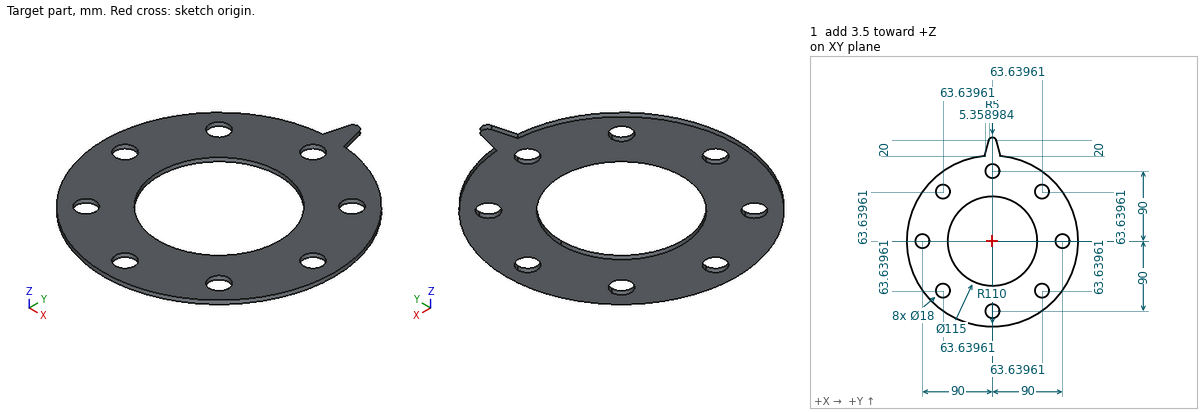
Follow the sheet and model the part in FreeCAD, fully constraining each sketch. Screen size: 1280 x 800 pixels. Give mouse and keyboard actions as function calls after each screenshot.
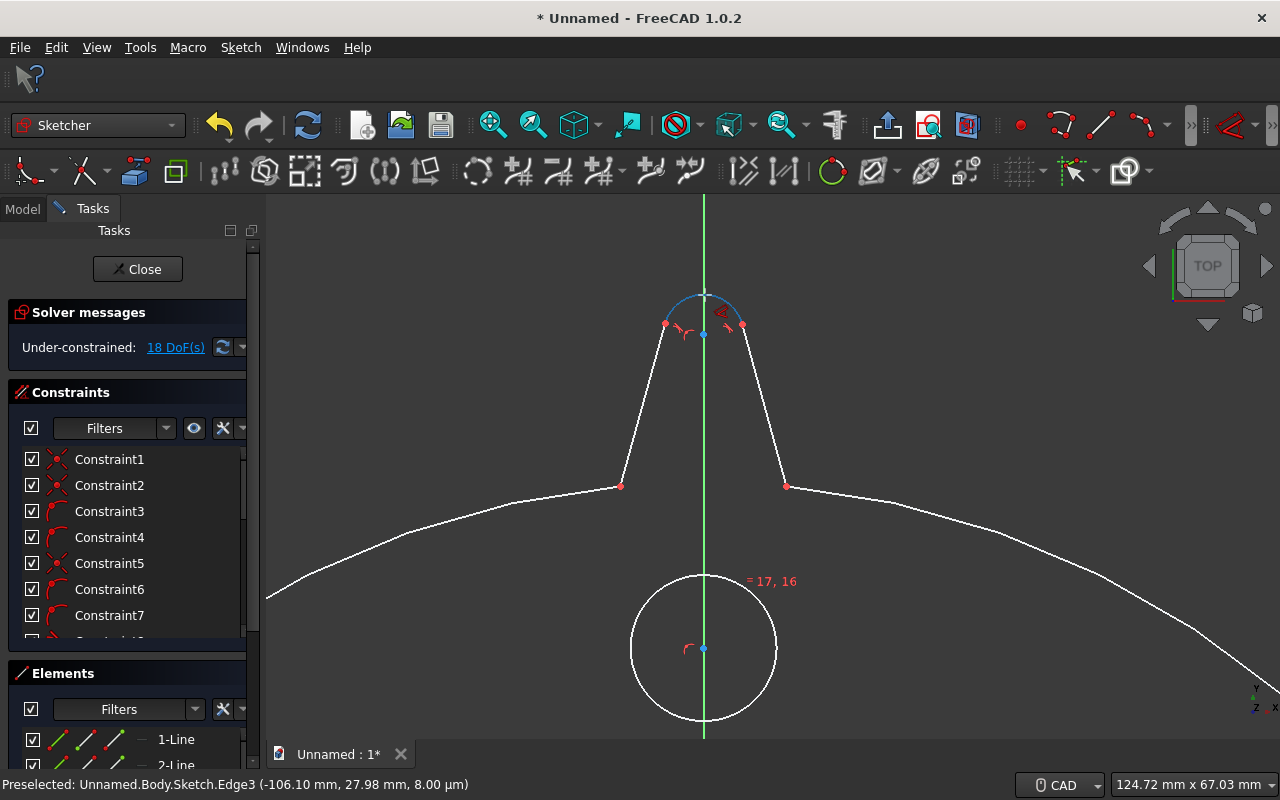
click(704, 295)
click(739, 272)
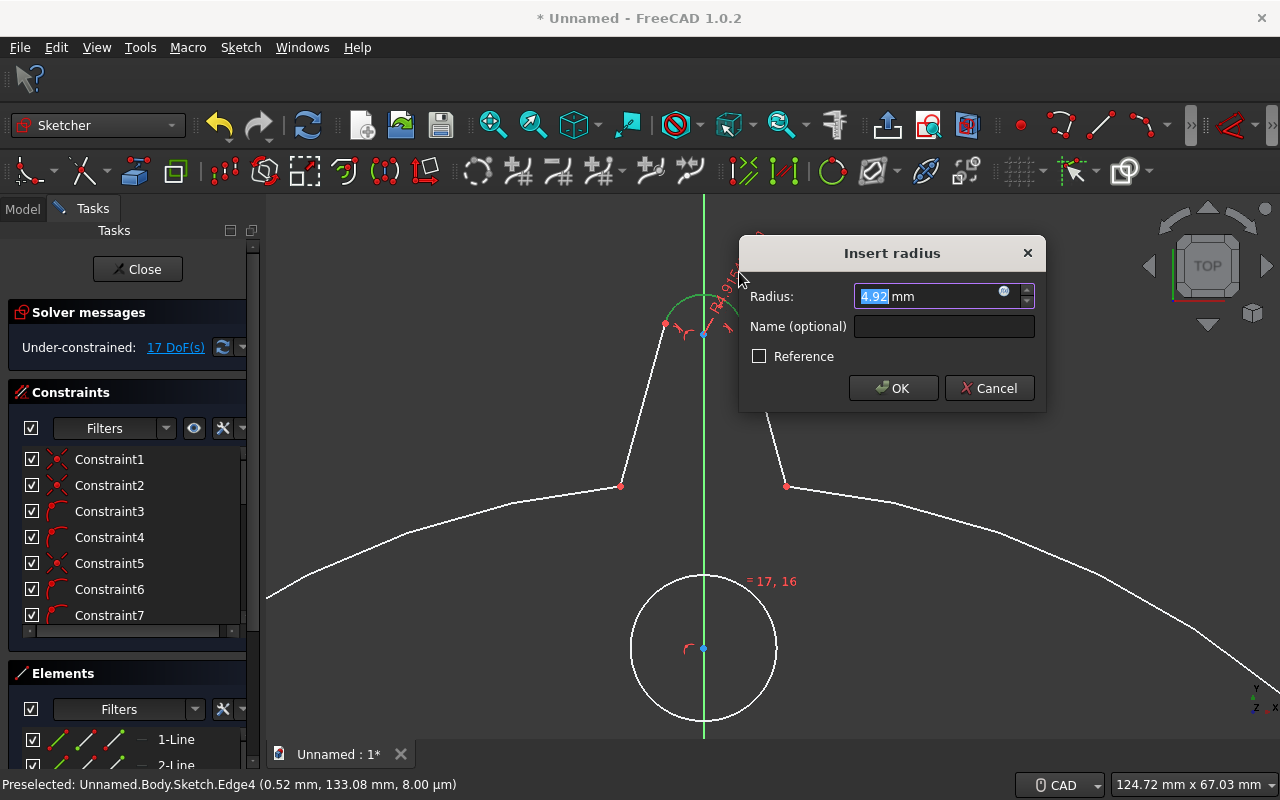
text(5)
key(Return)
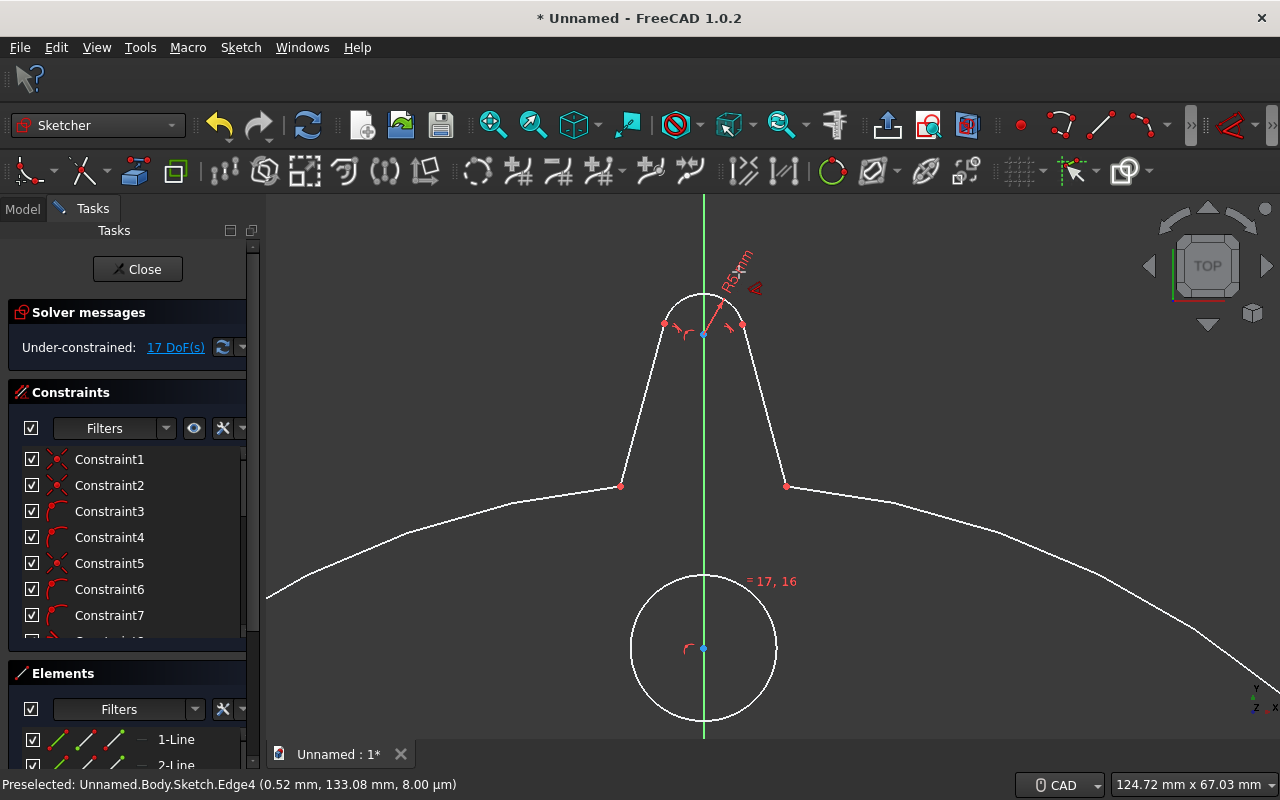
scroll(705, 305, down, 9)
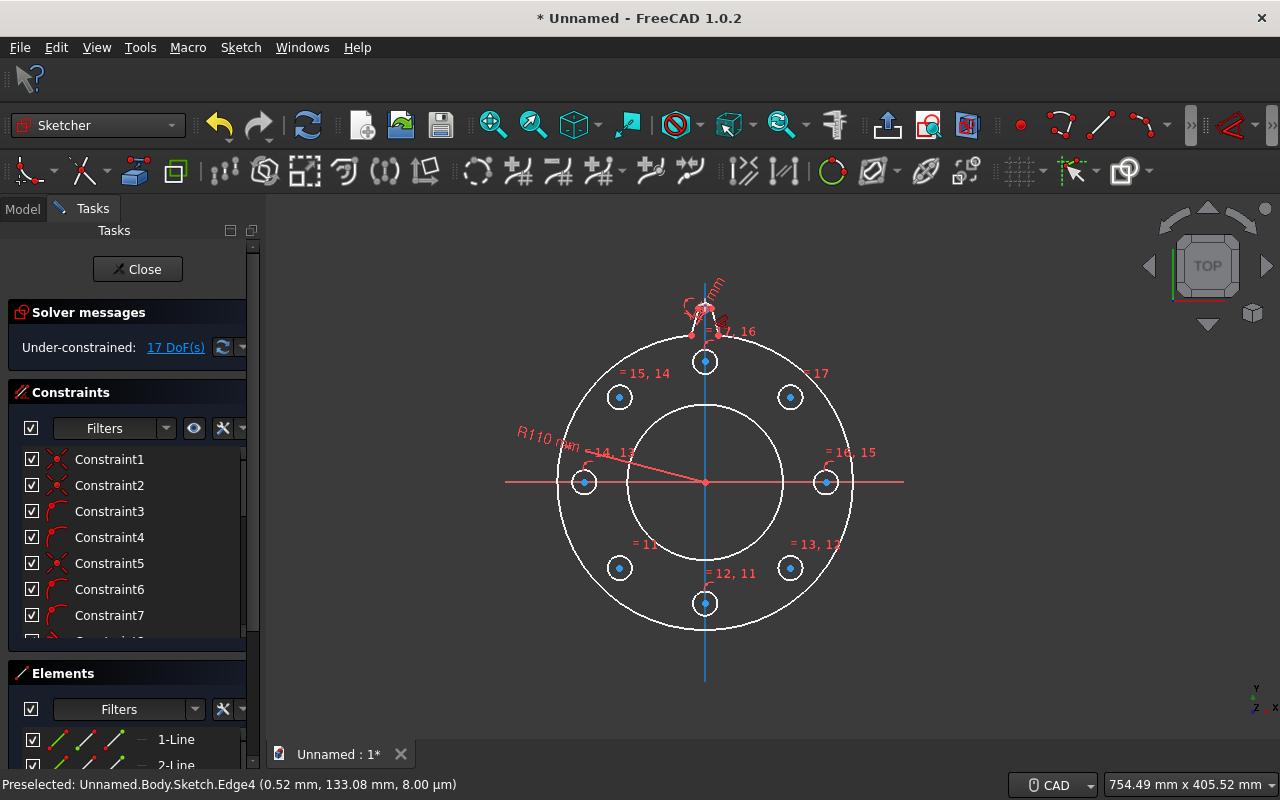
scroll(628, 560, up, 3)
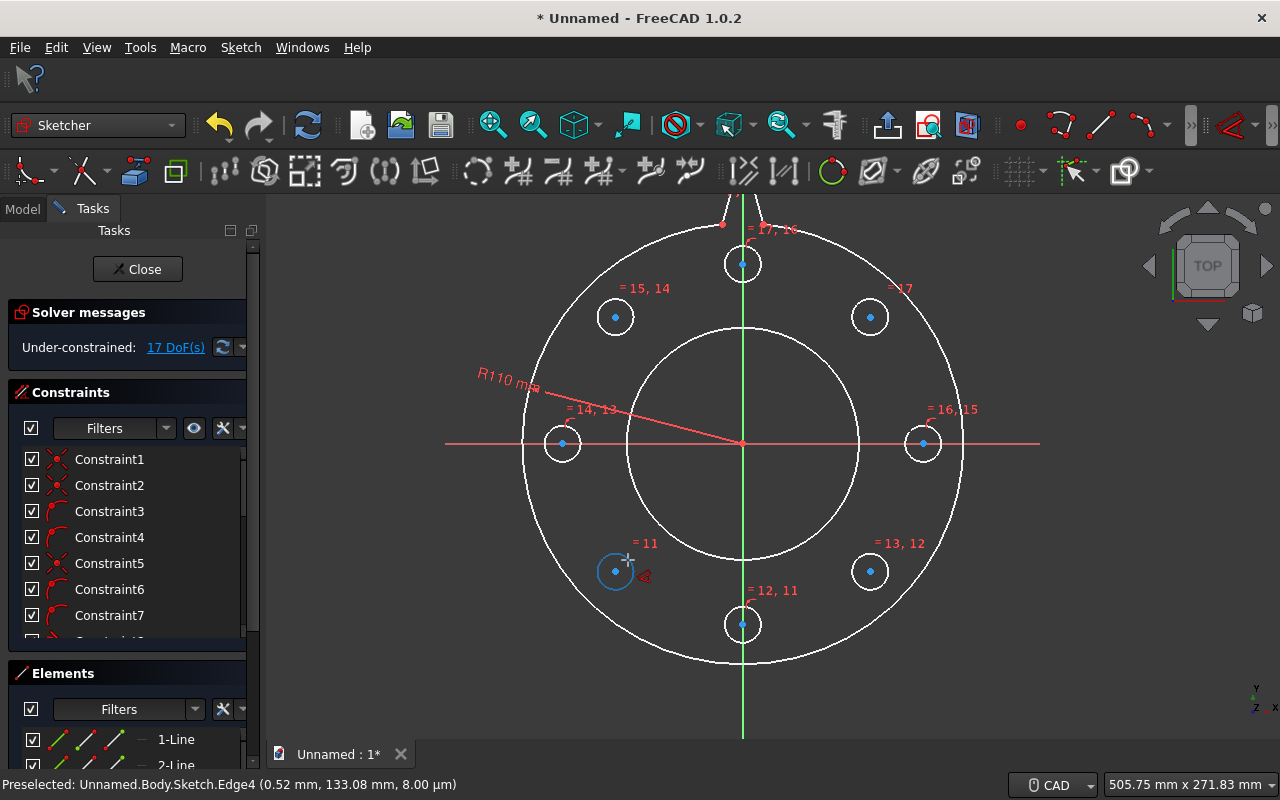
click(628, 559)
click(651, 536)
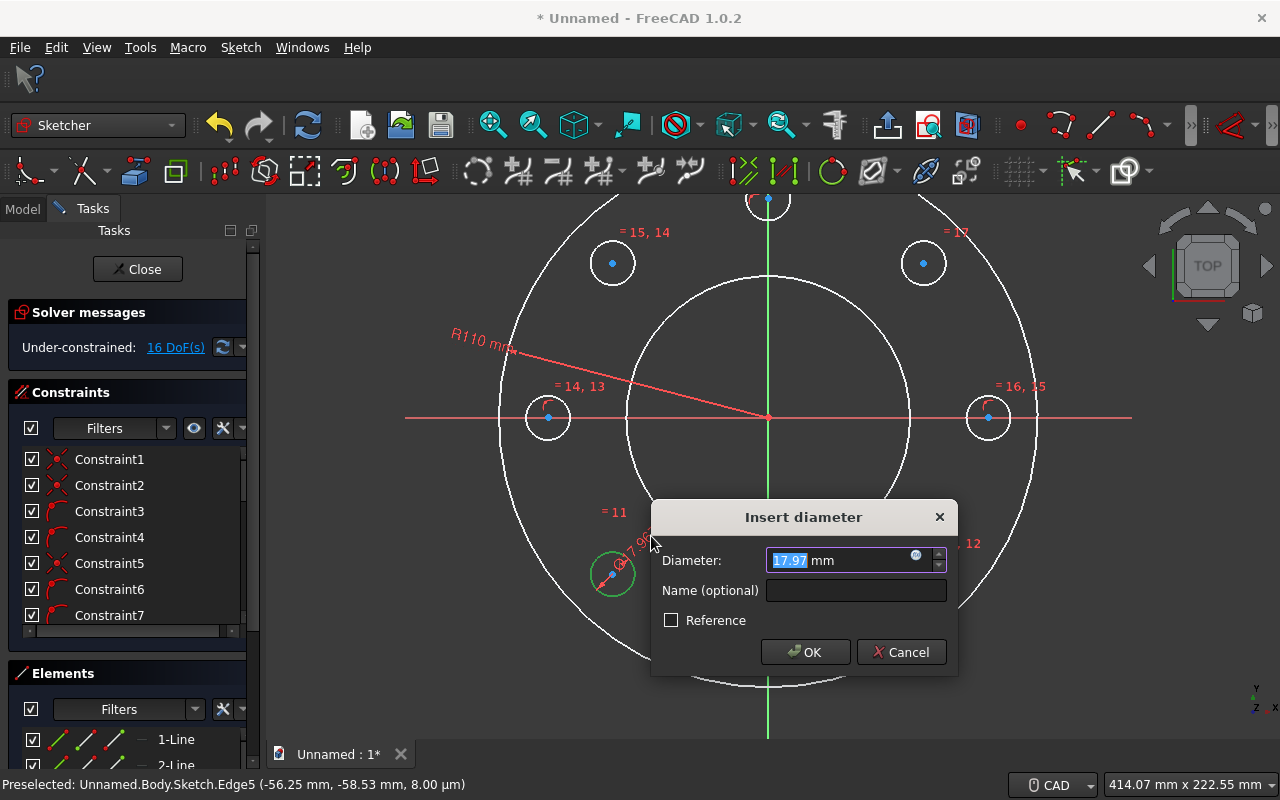
text(18)
key(Return)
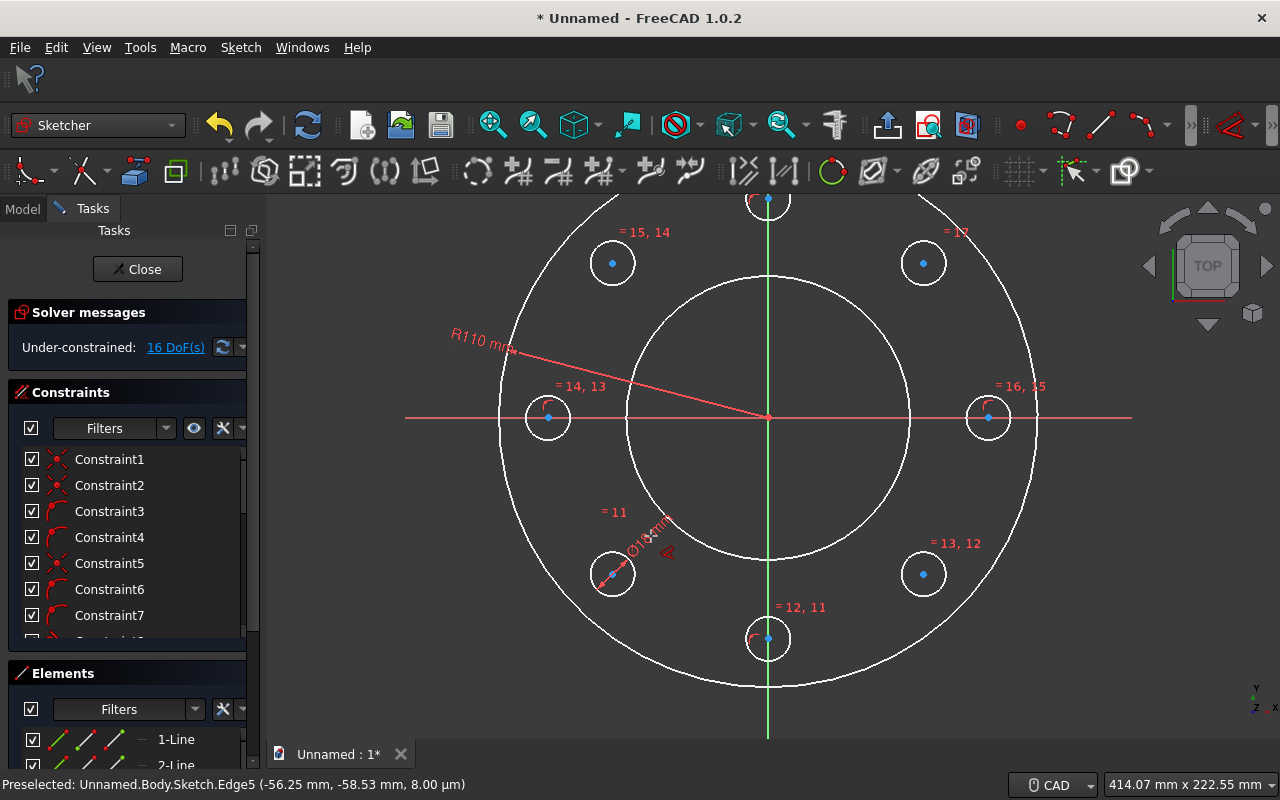
click(868, 317)
click(890, 294)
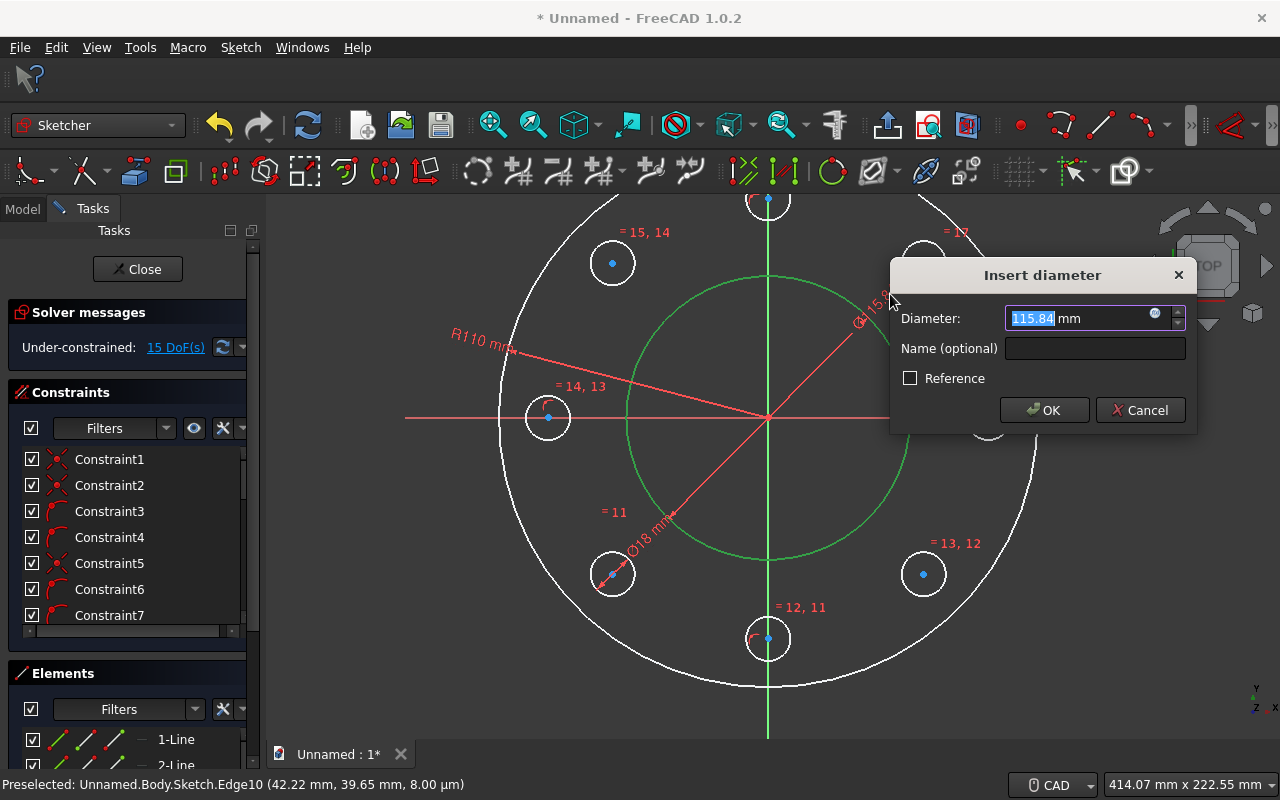
text(115)
key(Return)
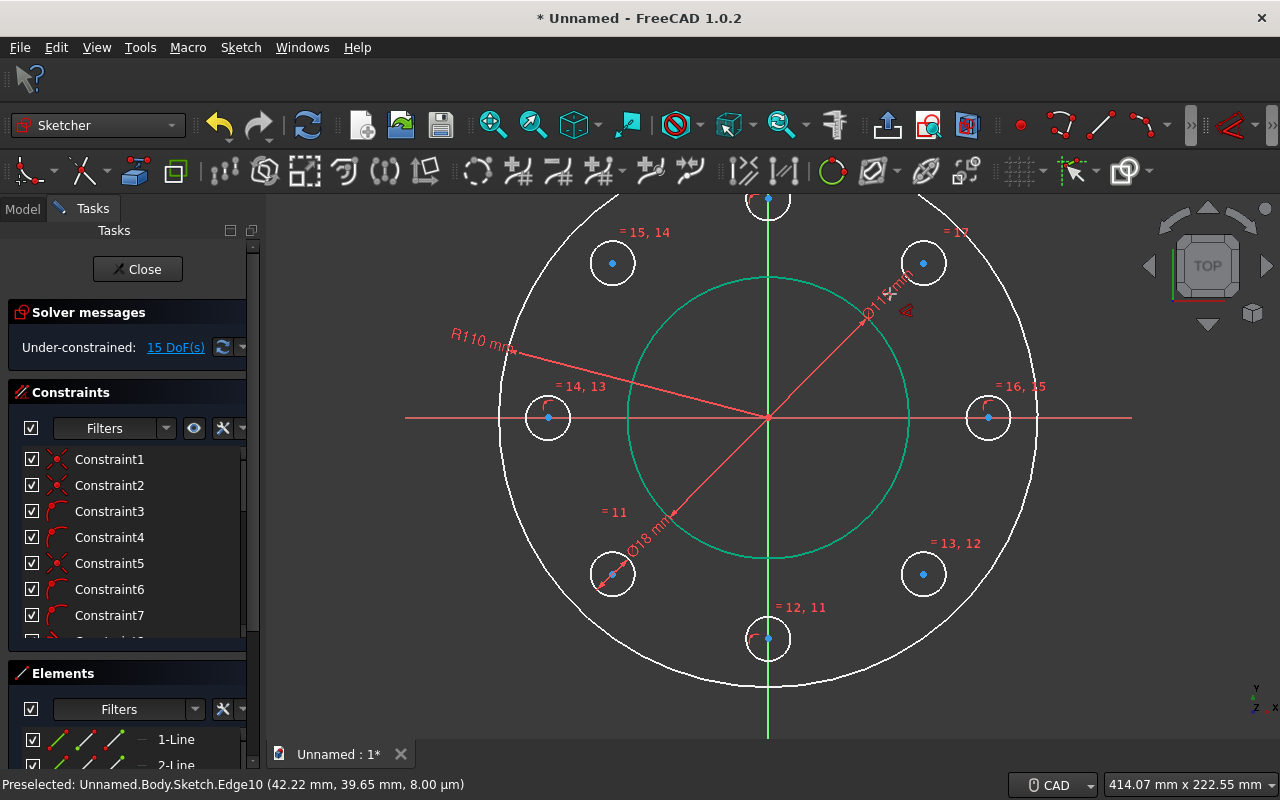
click(768, 639)
click(802, 528)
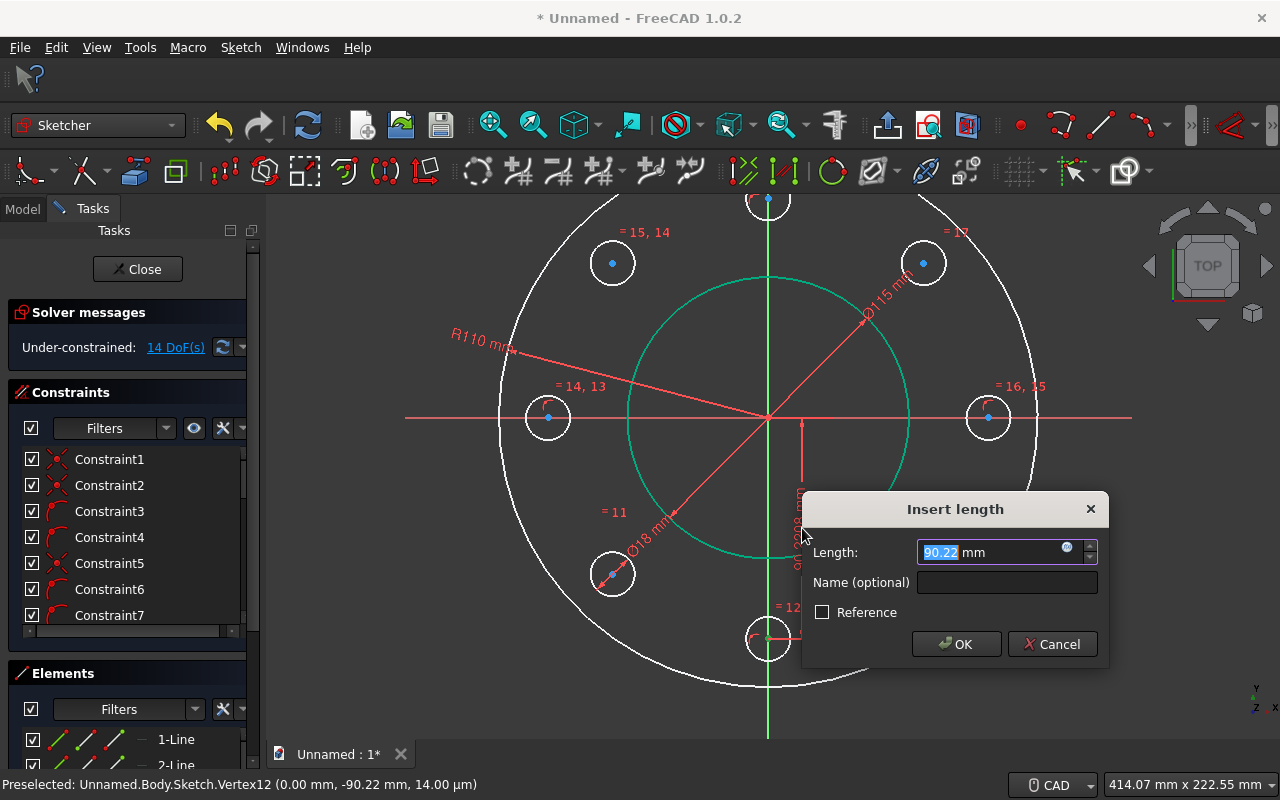
text(90)
key(Return)